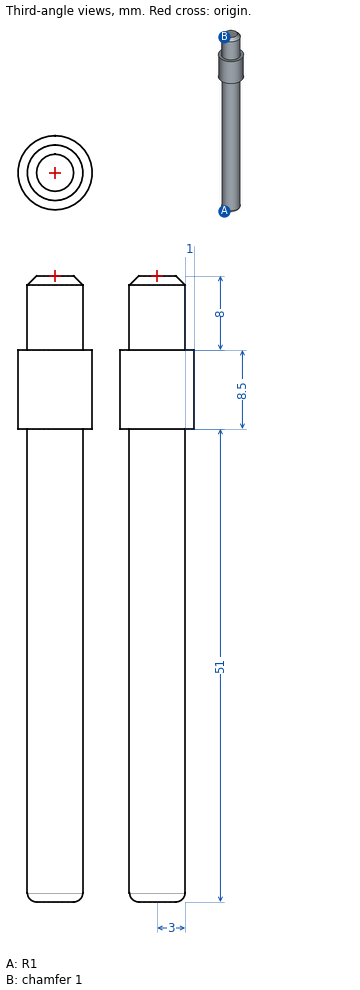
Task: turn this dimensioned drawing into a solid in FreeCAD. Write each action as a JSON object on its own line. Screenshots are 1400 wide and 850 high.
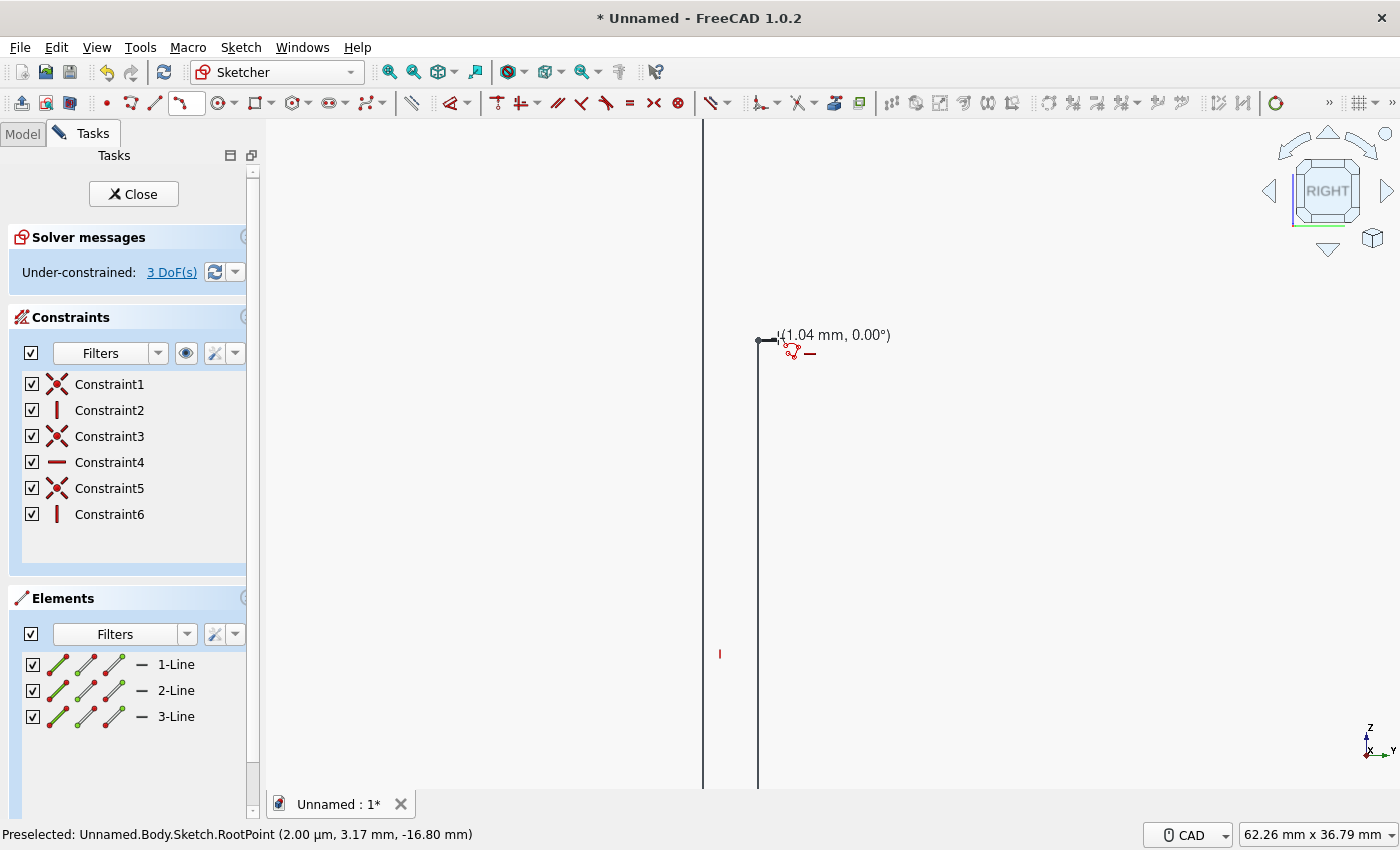
{"action": "left_click", "coordinate": [776, 337]}
{"action": "left_click", "coordinate": [776, 183]}
{"action": "left_click", "coordinate": [758, 183]}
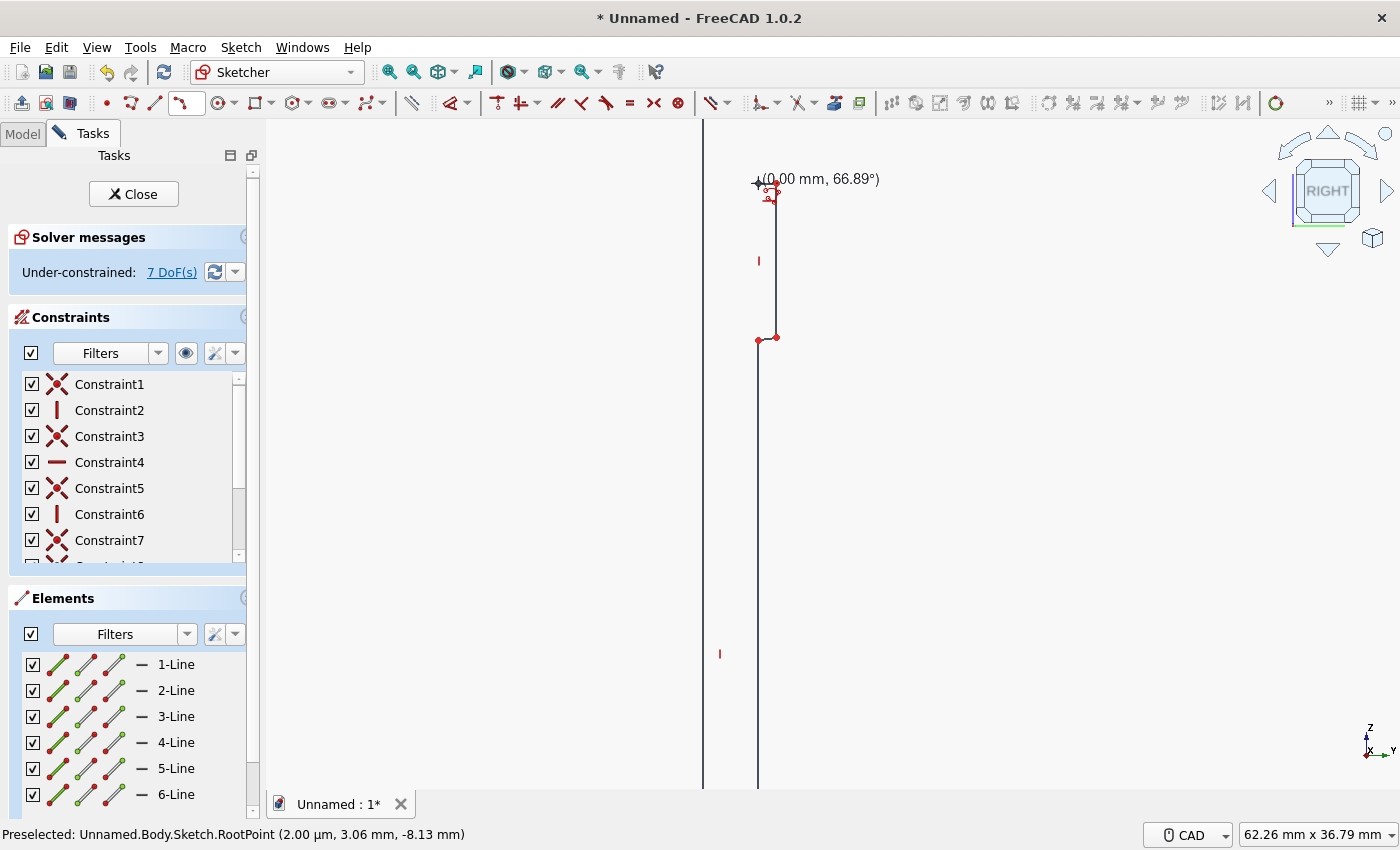
{"action": "scroll", "coordinate": [779, 339], "scroll_direction": "down", "scroll_amount": 5}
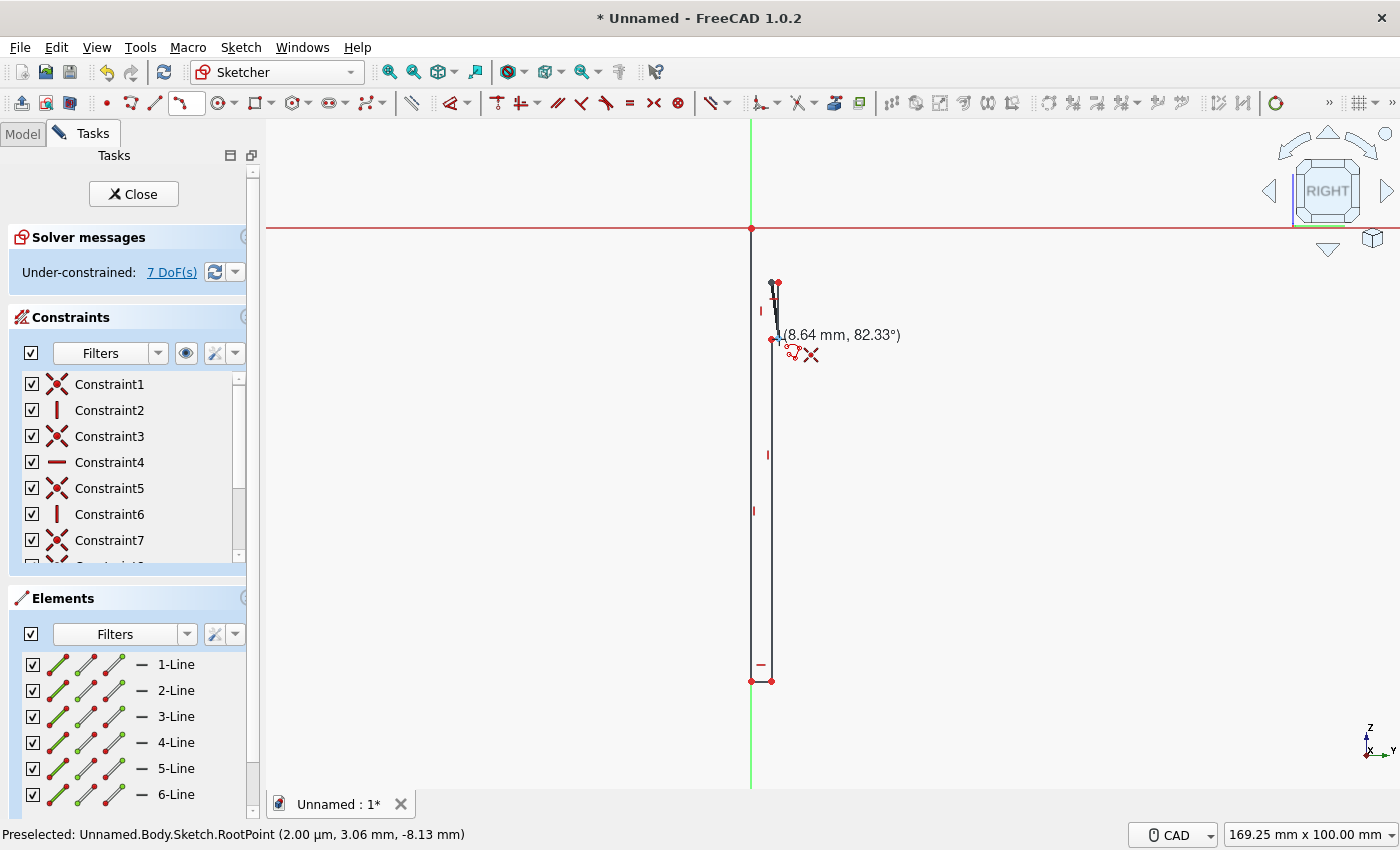
{"action": "left_click", "coordinate": [772, 237]}
{"action": "left_click", "coordinate": [751, 228]}
{"action": "key", "text": "Escape"}
{"action": "key", "text": "Escape"}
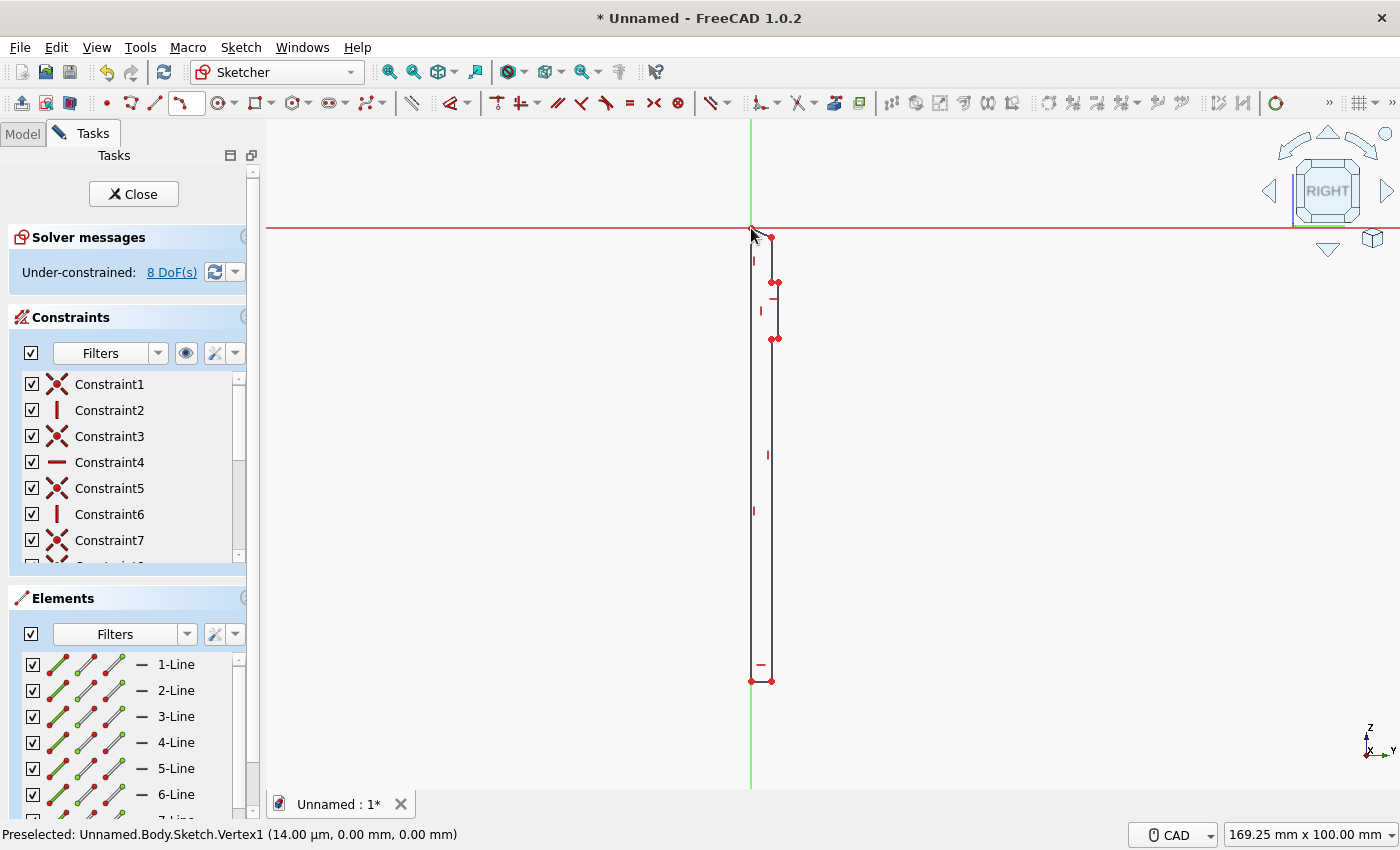
{"action": "scroll", "coordinate": [775, 339], "scroll_direction": "up", "scroll_amount": 8}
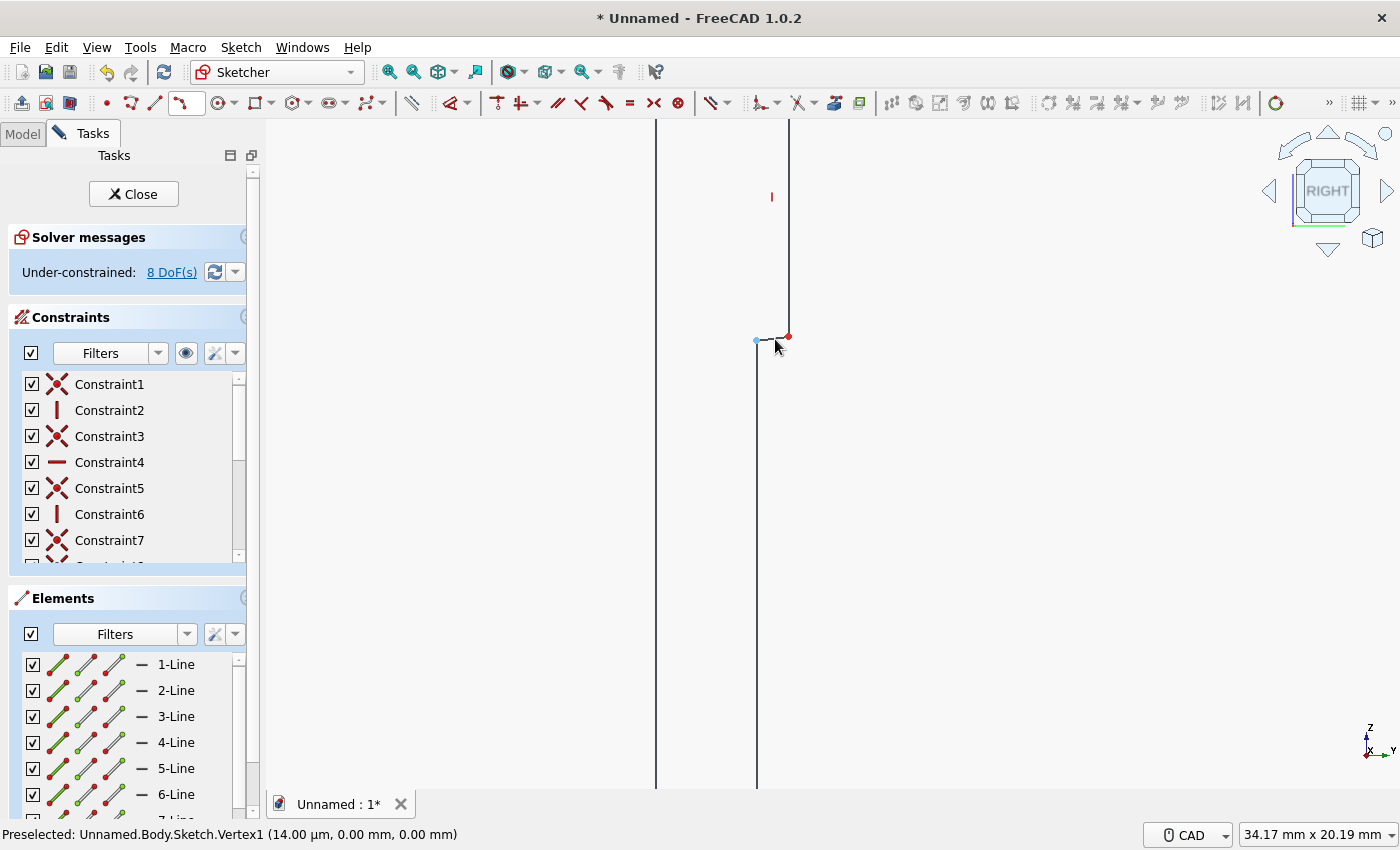
{"action": "left_click", "coordinate": [773, 339]}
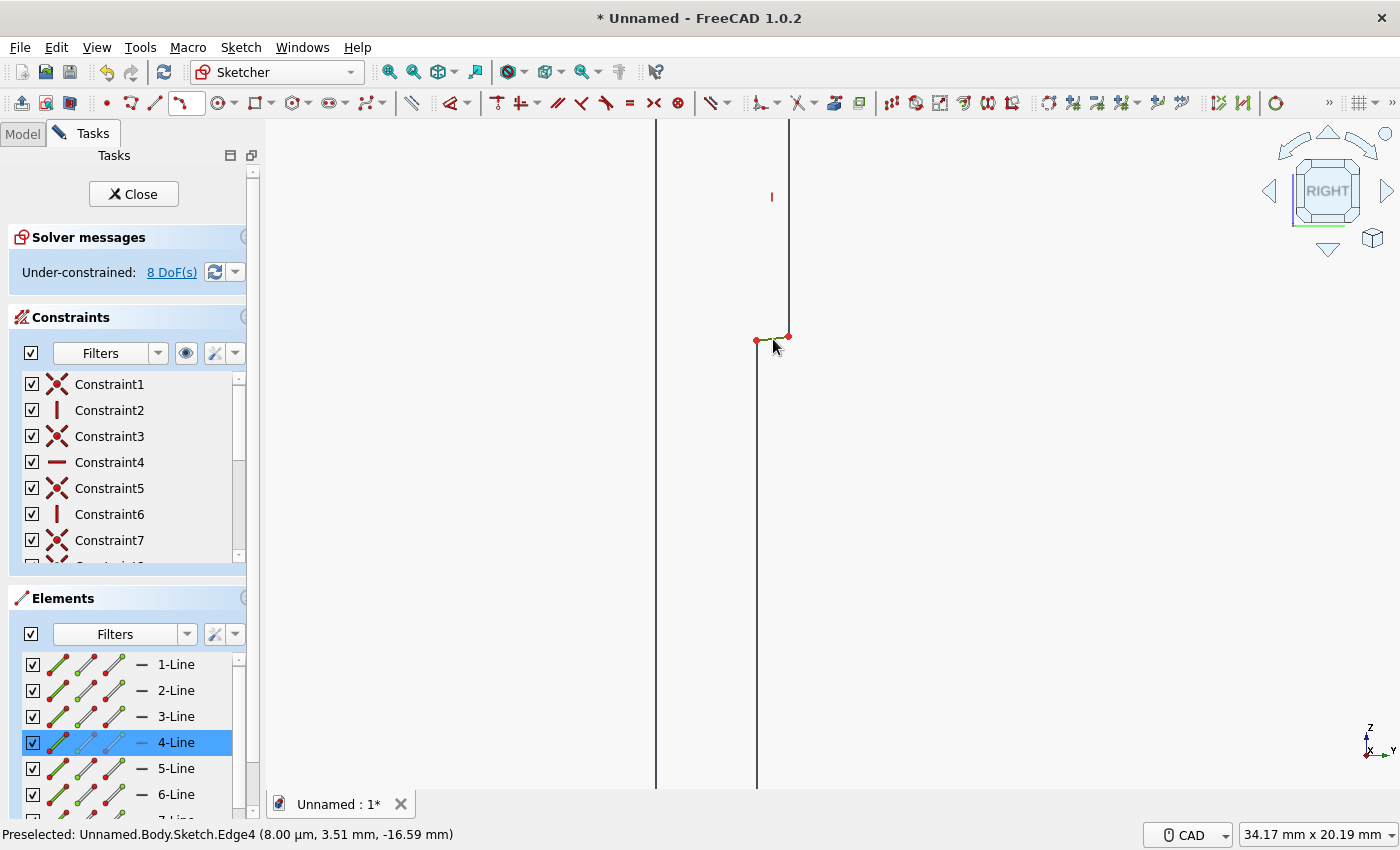
{"action": "left_click", "coordinate": [540, 104]}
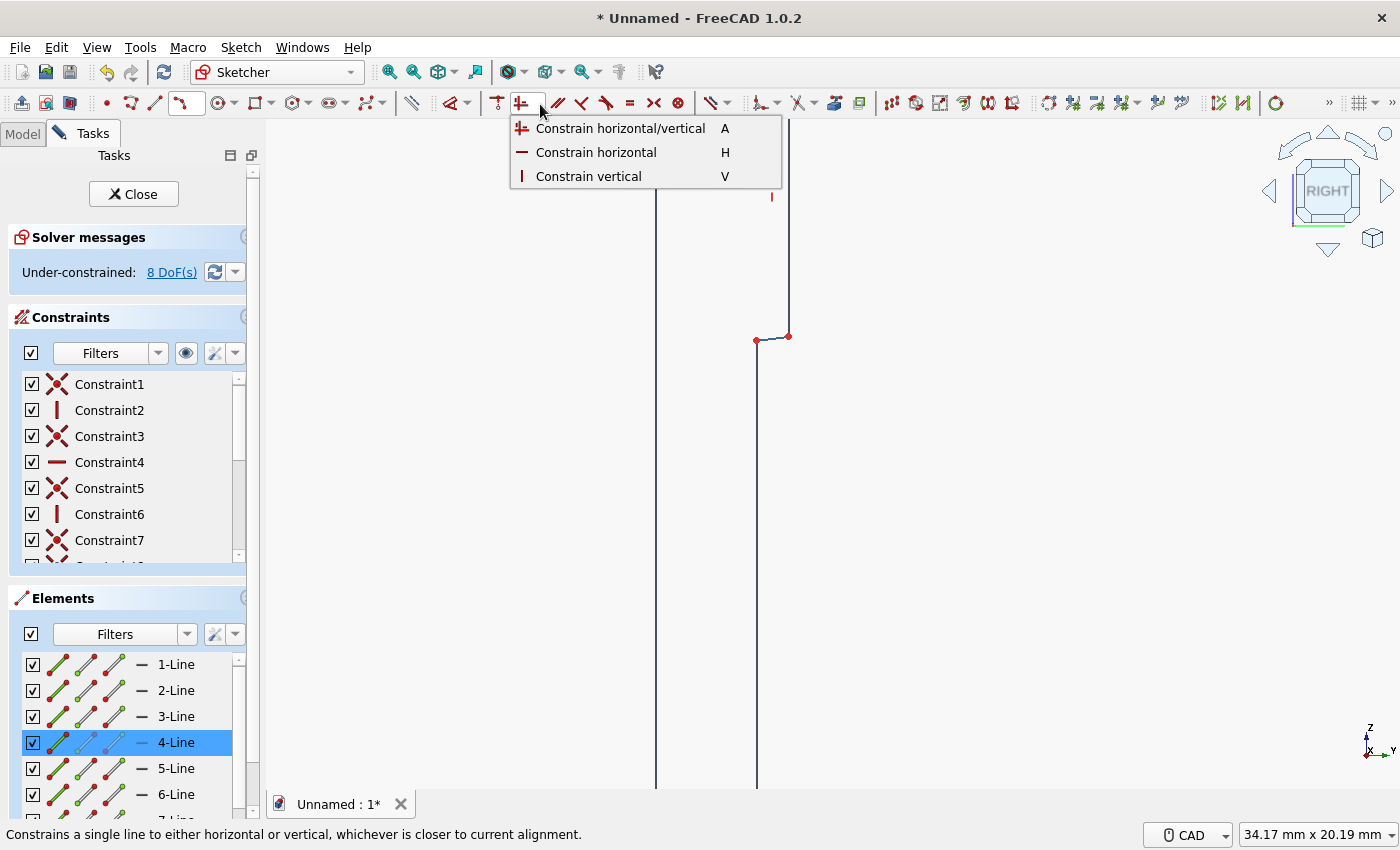
{"action": "left_click", "coordinate": [646, 152]}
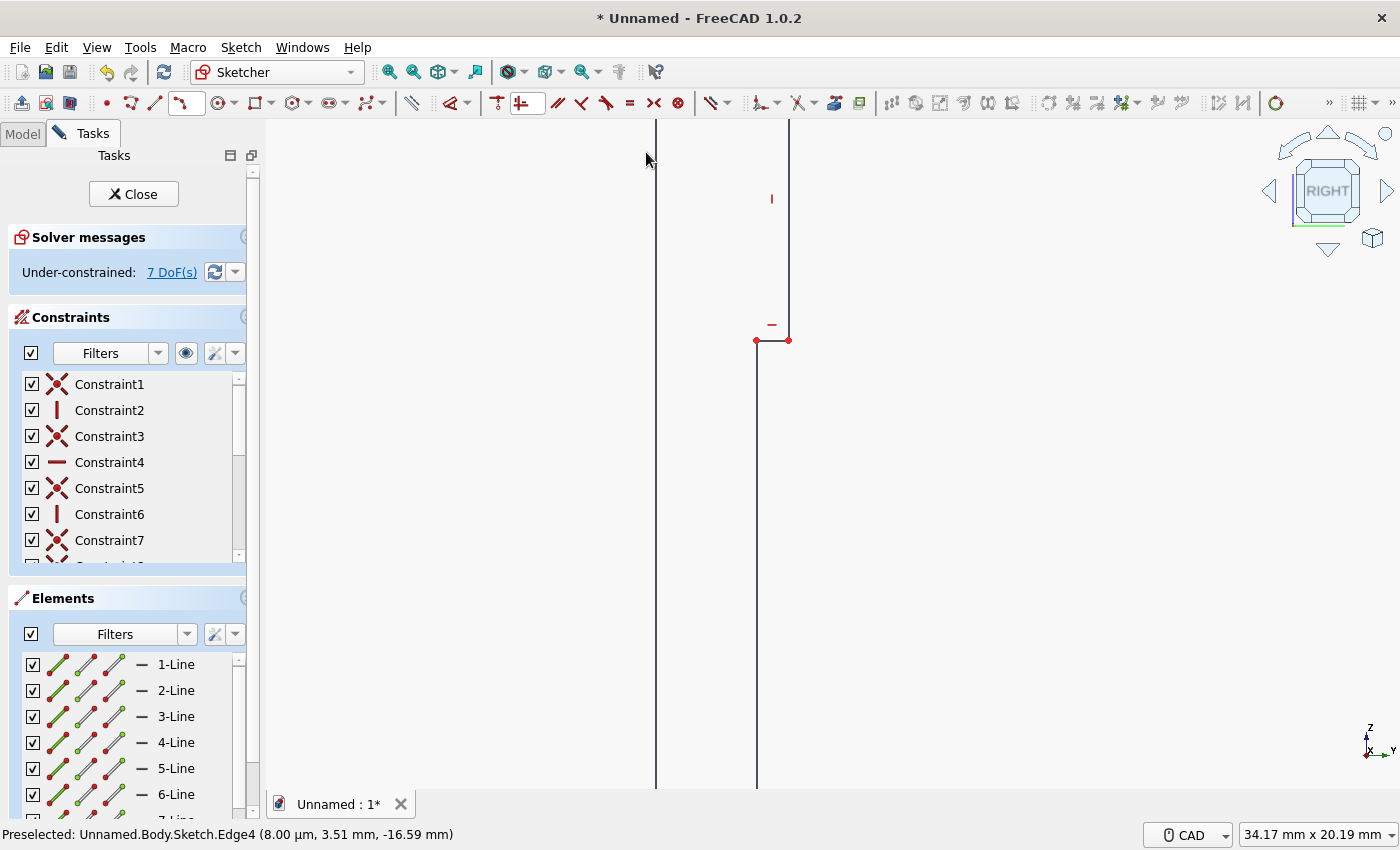
{"action": "scroll", "coordinate": [775, 339], "scroll_direction": "down", "scroll_amount": 8}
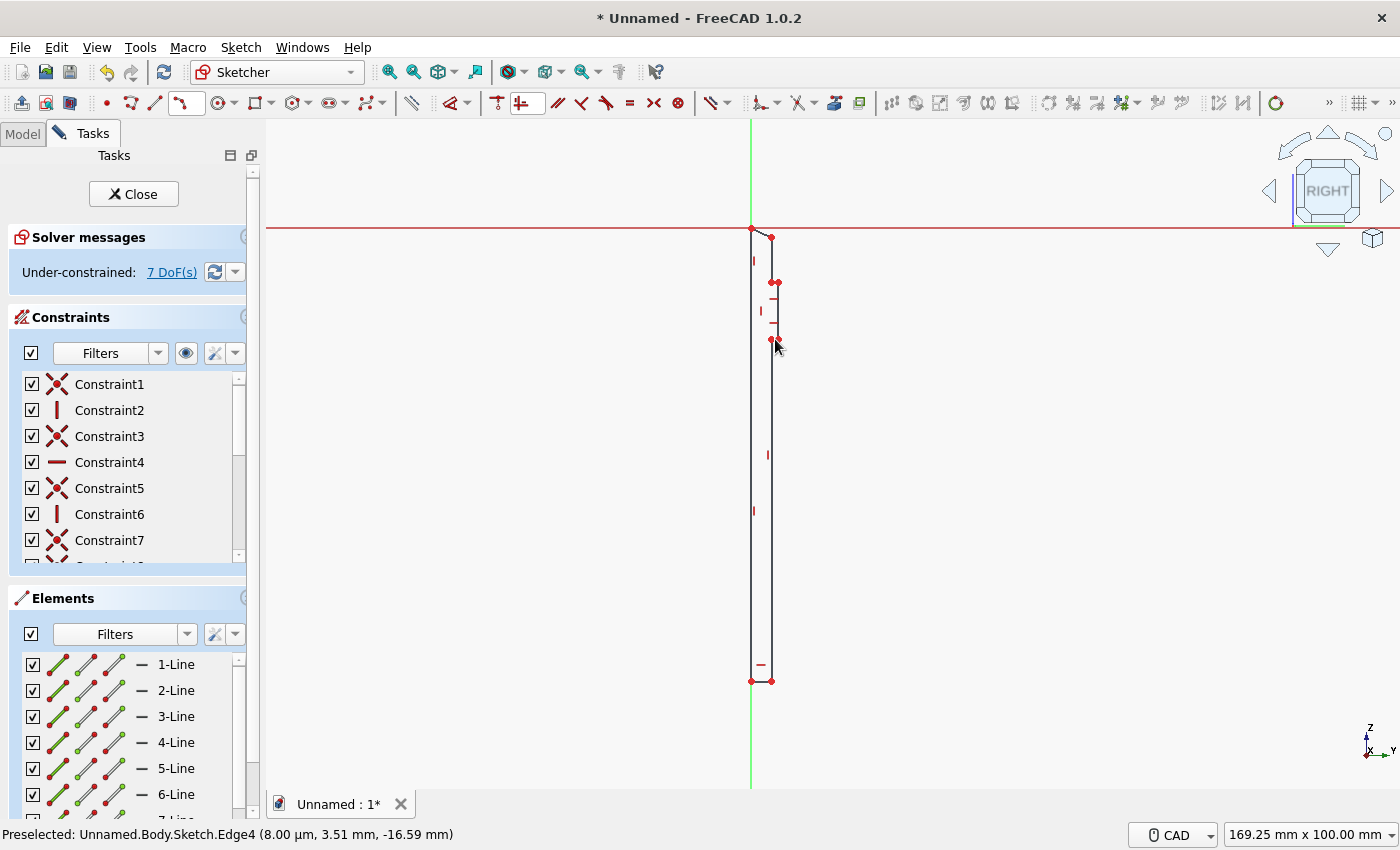
{"action": "scroll", "coordinate": [766, 235], "scroll_direction": "up", "scroll_amount": 4}